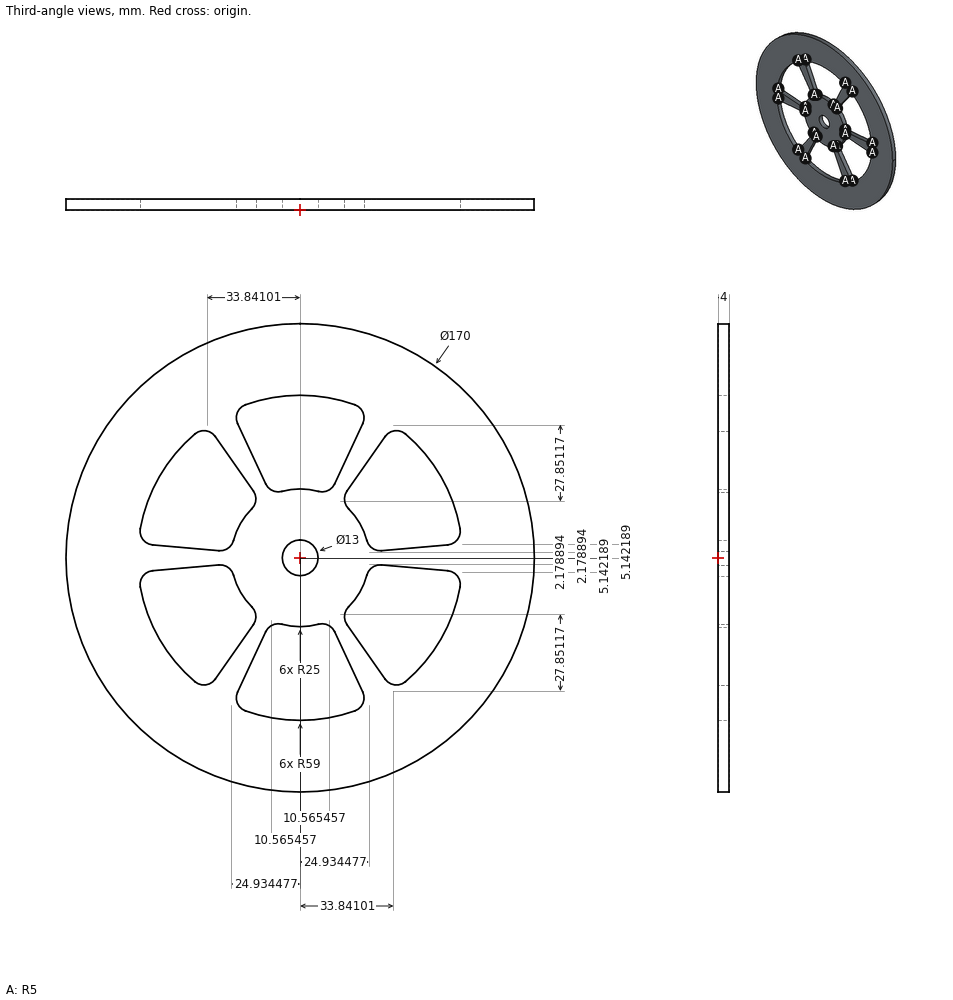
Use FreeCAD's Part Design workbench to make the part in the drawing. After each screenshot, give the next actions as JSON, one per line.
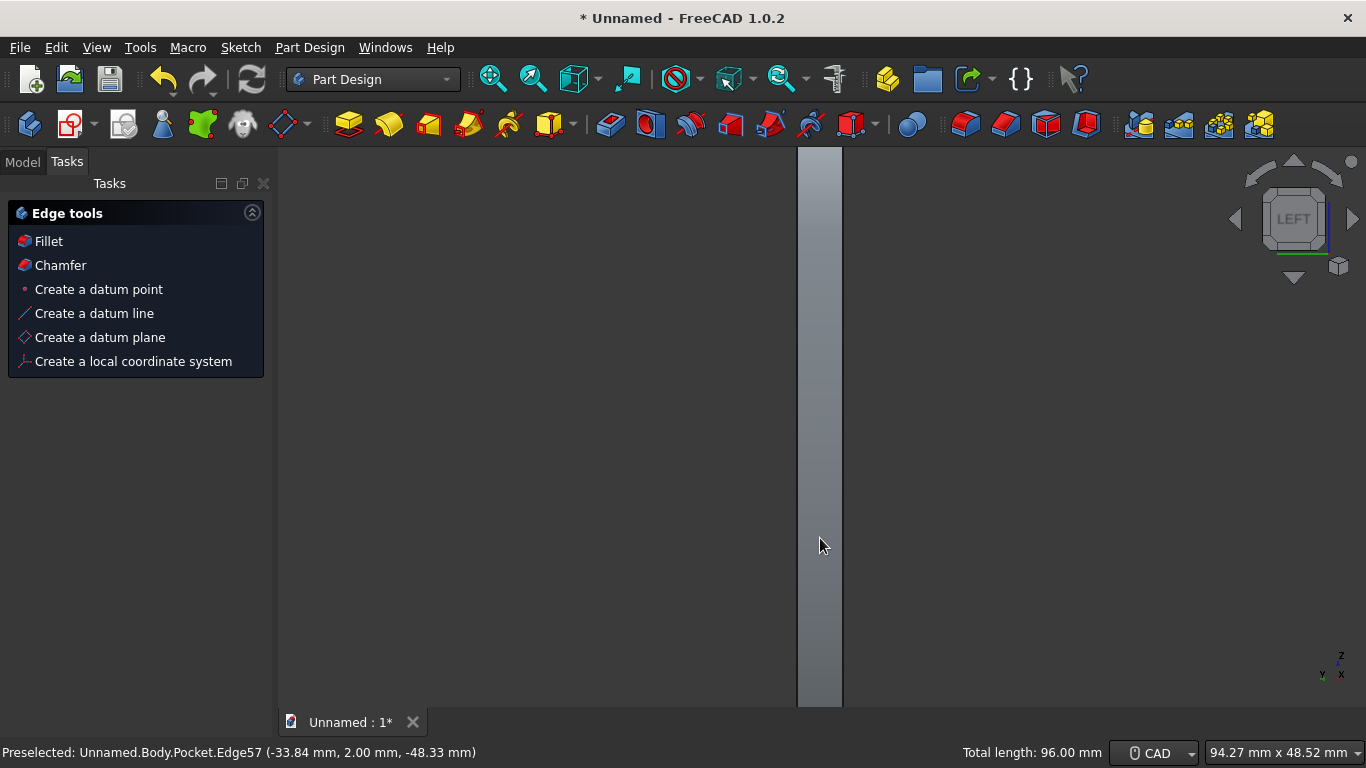
{"action": "left_click", "coordinate": [966, 124]}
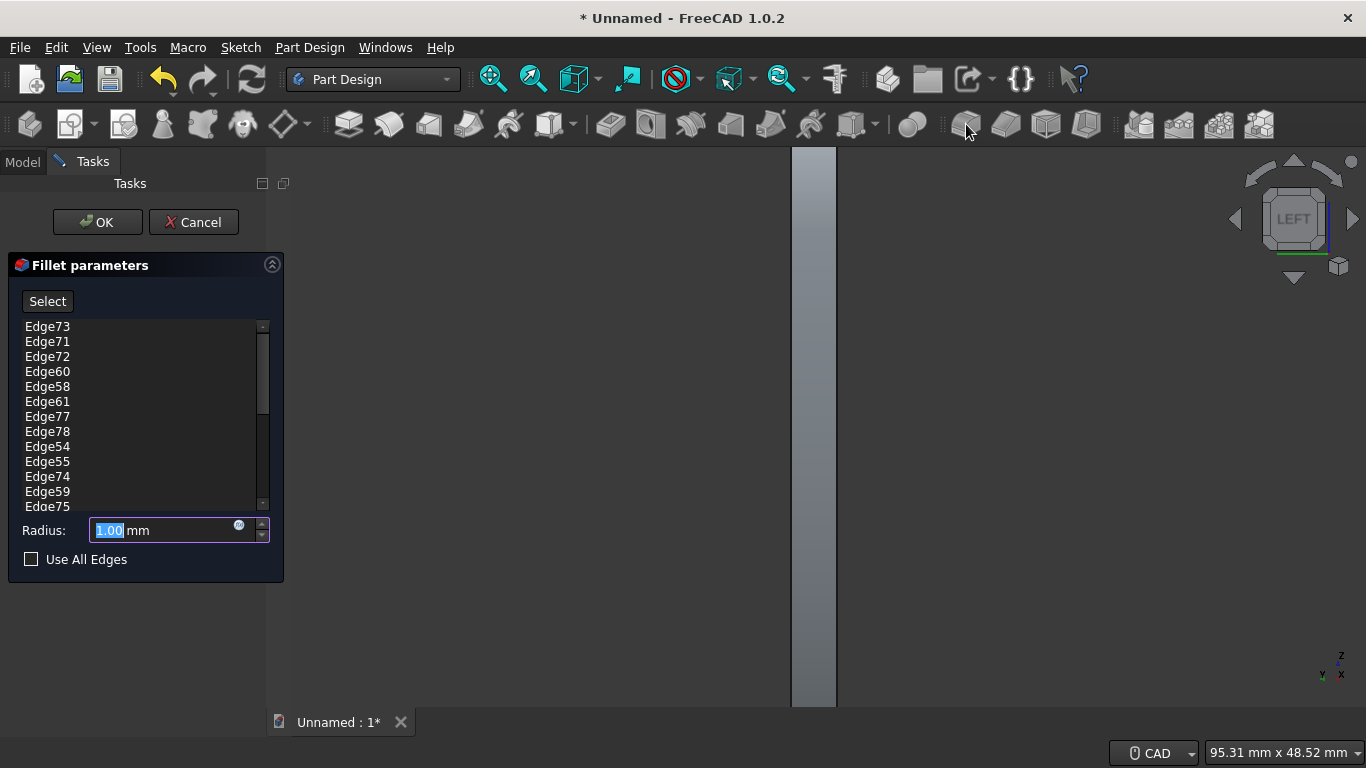
{"action": "type", "text": "5"}
{"action": "key", "text": "Tab"}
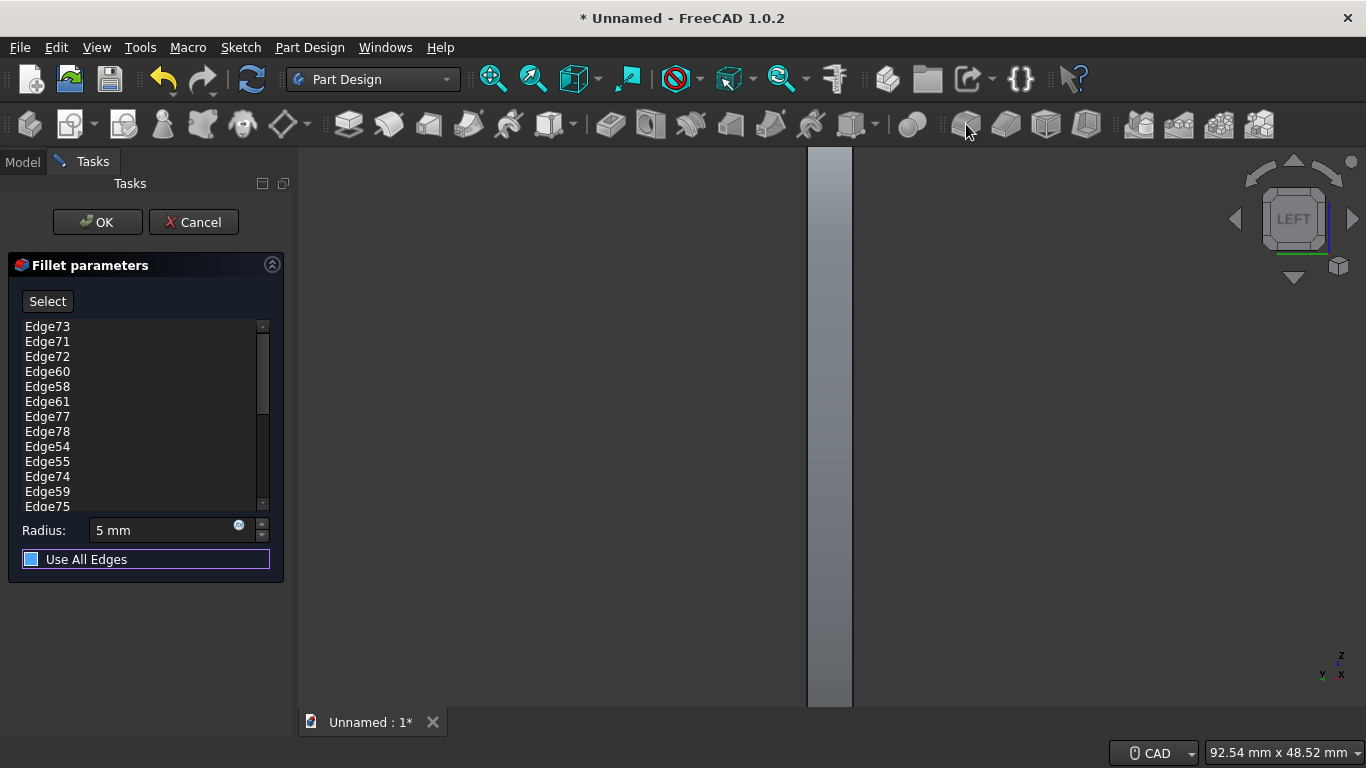
{"action": "left_click", "coordinate": [98, 222]}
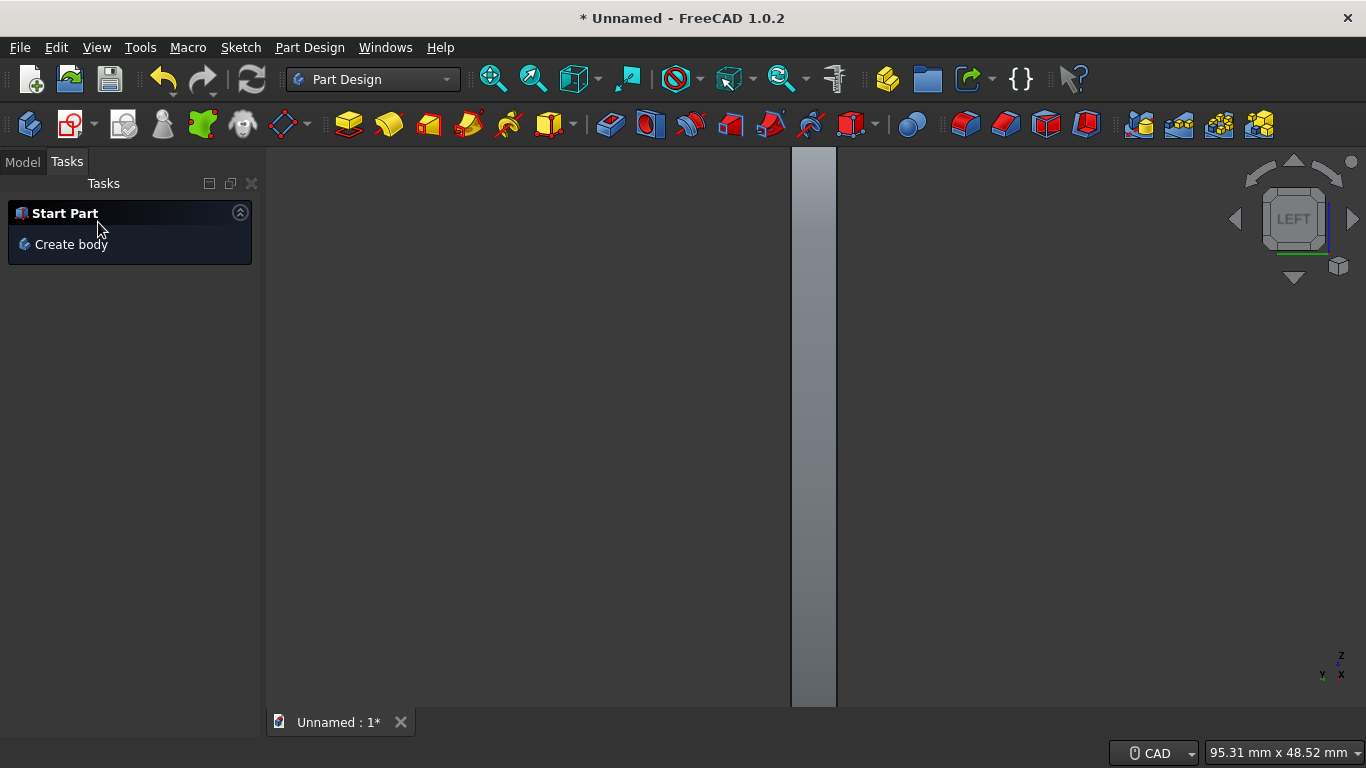
{"action": "key", "text": "0"}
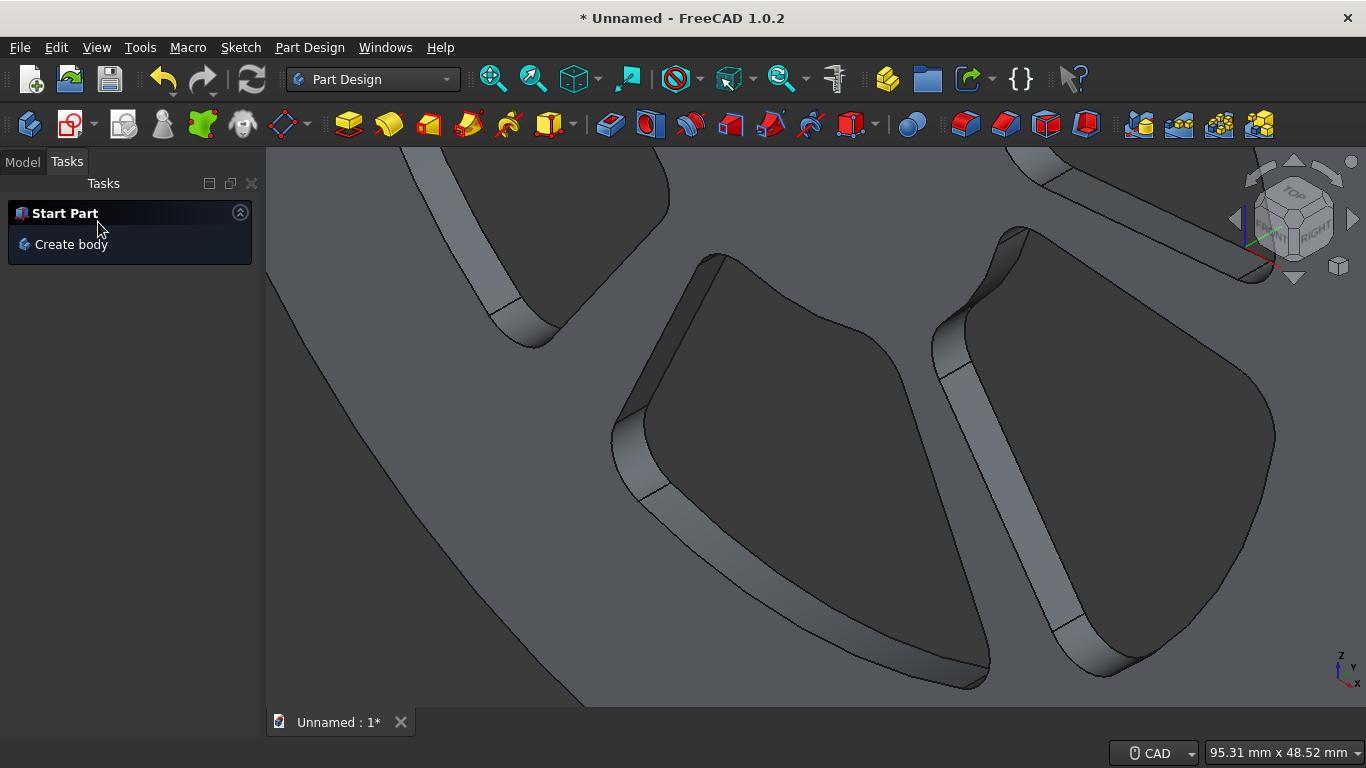
{"action": "left_click", "coordinate": [494, 80]}